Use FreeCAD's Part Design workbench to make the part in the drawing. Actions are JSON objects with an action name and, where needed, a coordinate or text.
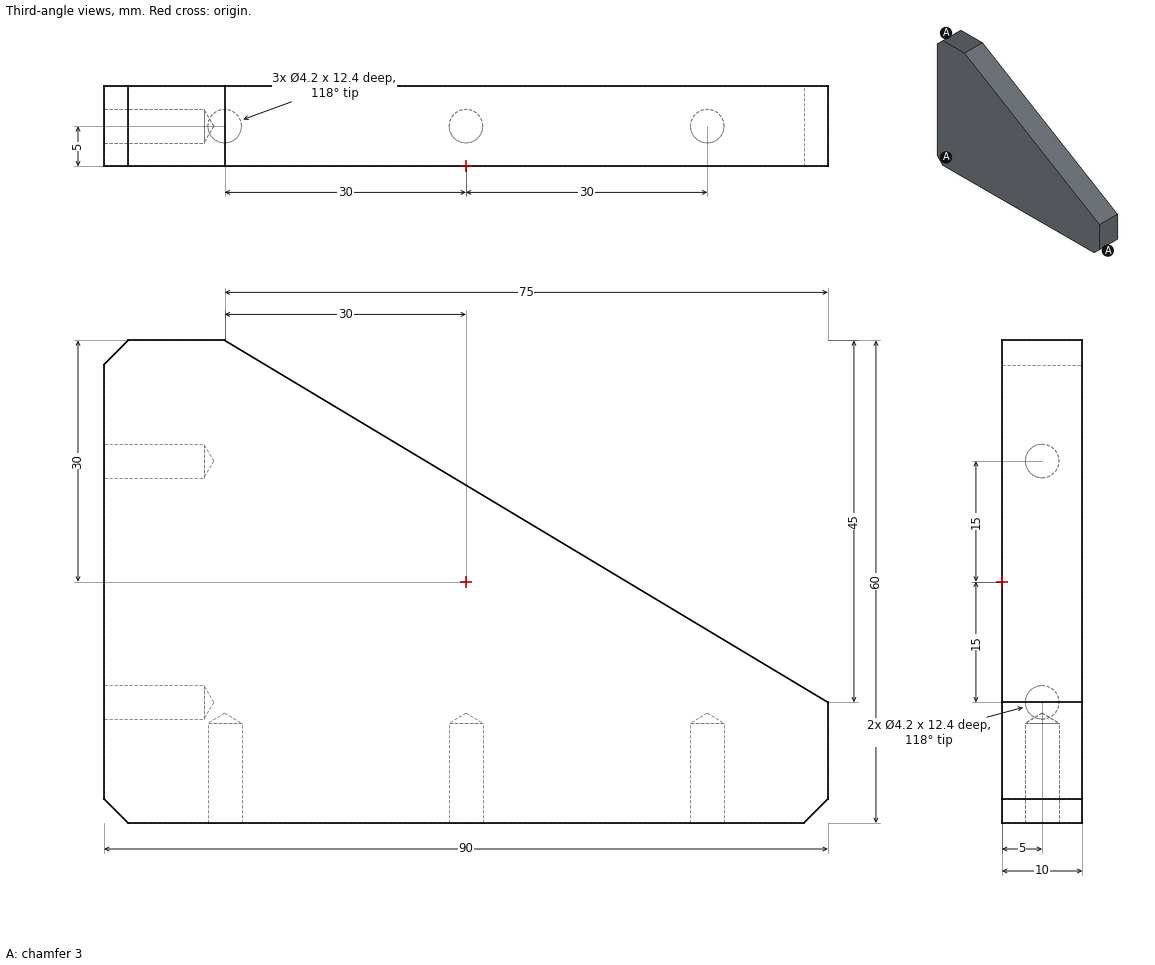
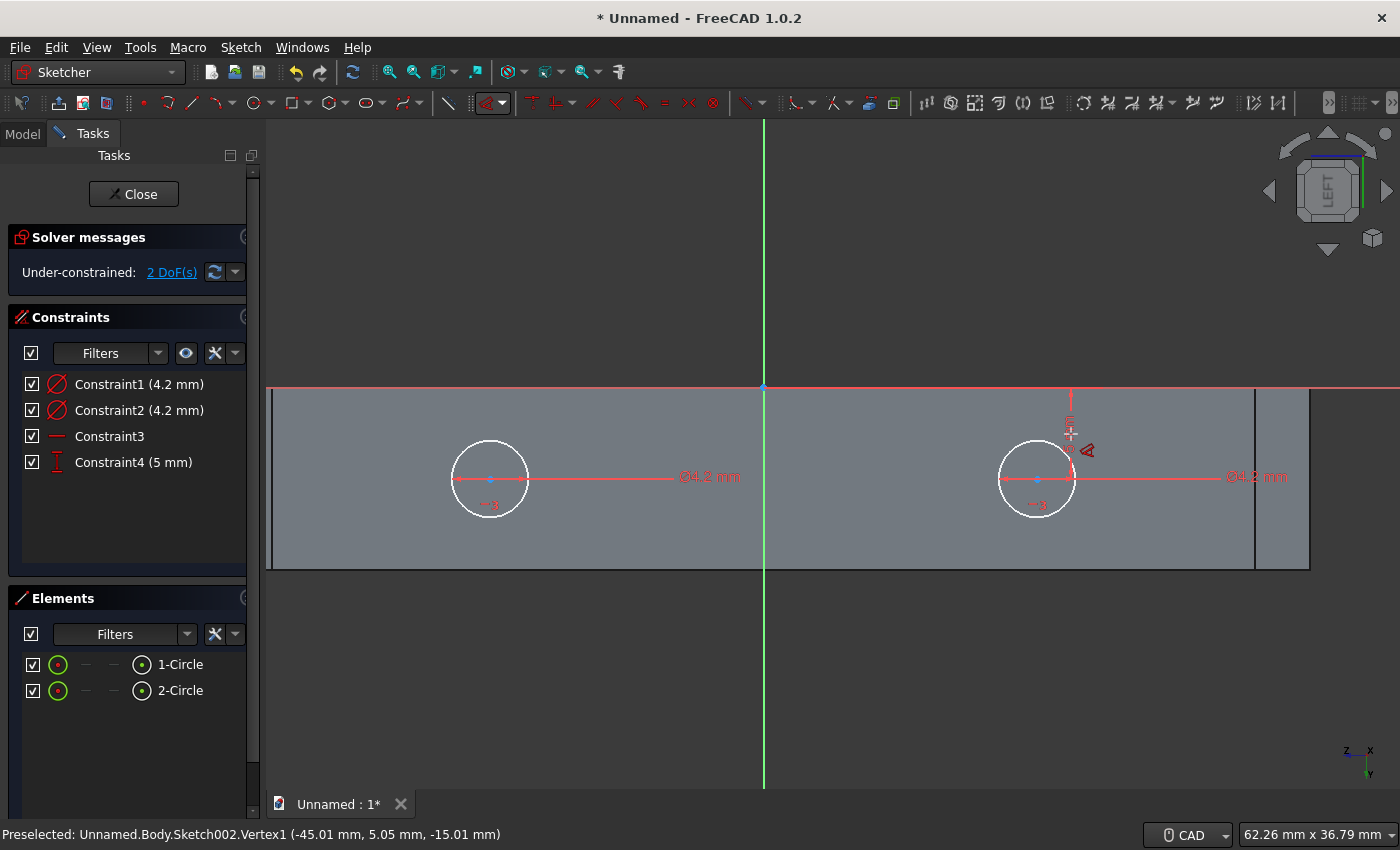
{"action": "left_click", "coordinate": [1037, 479]}
{"action": "left_click", "coordinate": [900, 354]}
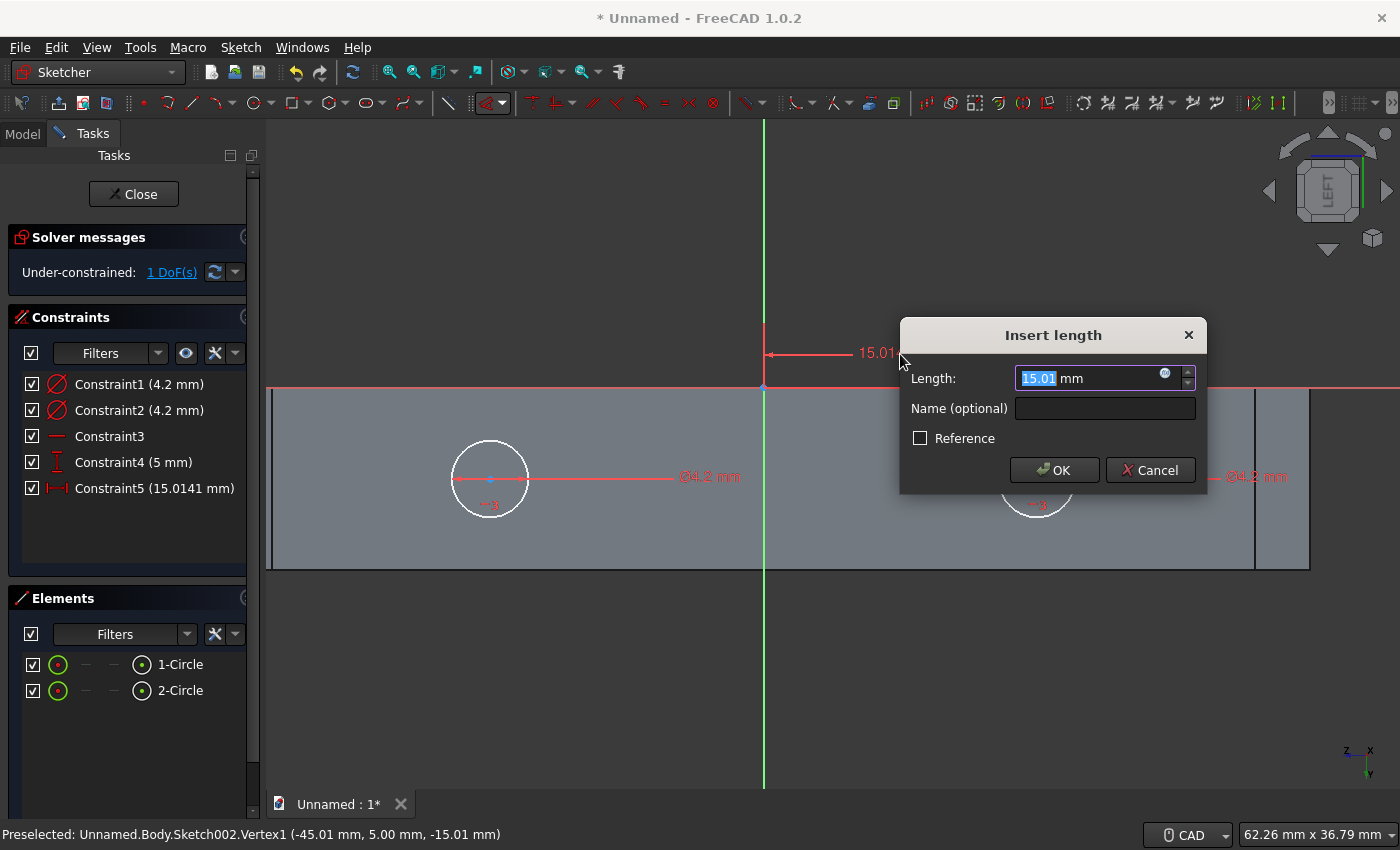
{"action": "type", "text": "15"}
{"action": "key", "text": "Return"}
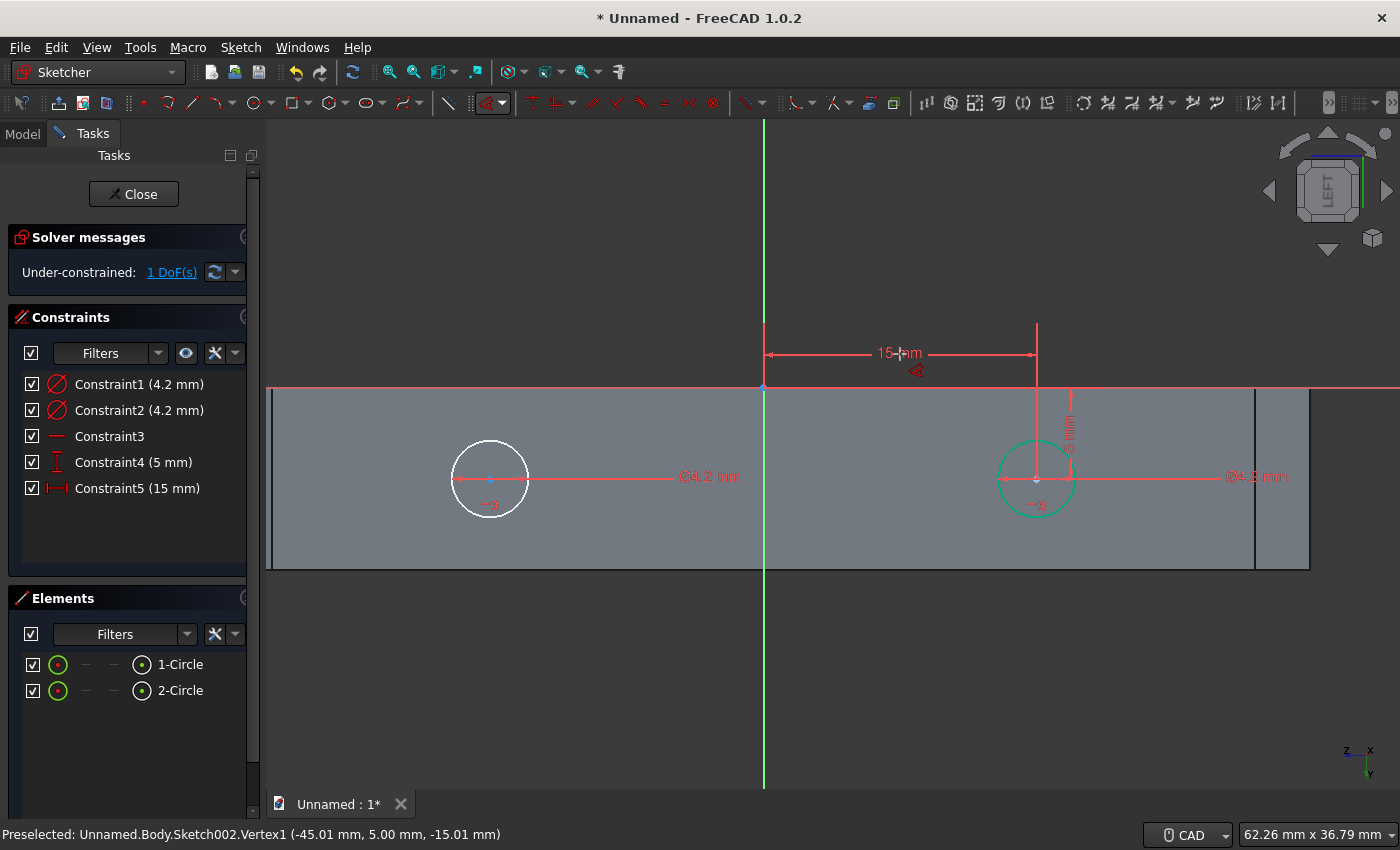
{"action": "left_click", "coordinate": [490, 479]}
{"action": "left_click", "coordinate": [627, 354]}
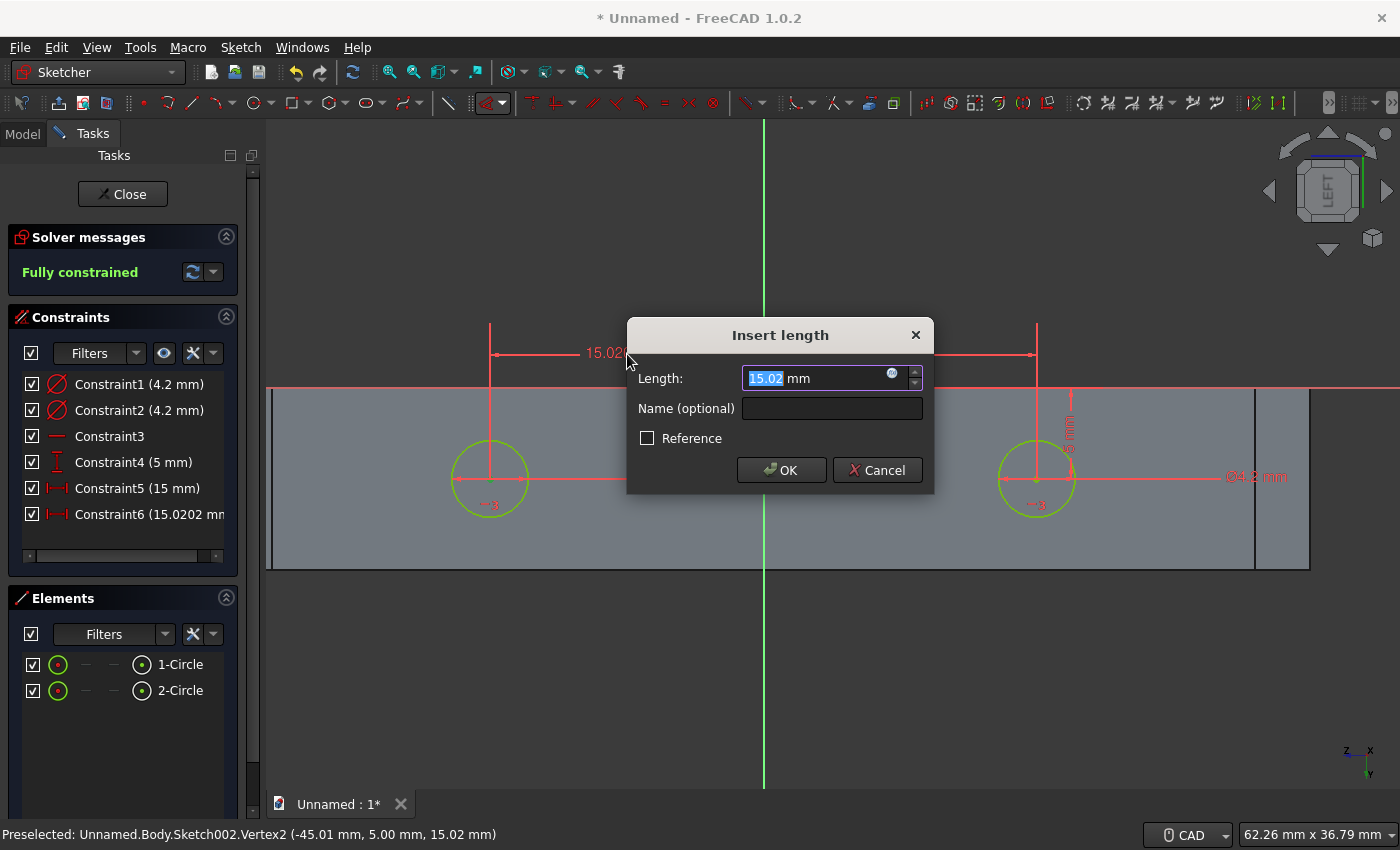
{"action": "type", "text": "15"}
{"action": "key", "text": "Return"}
{"action": "key", "text": "Escape"}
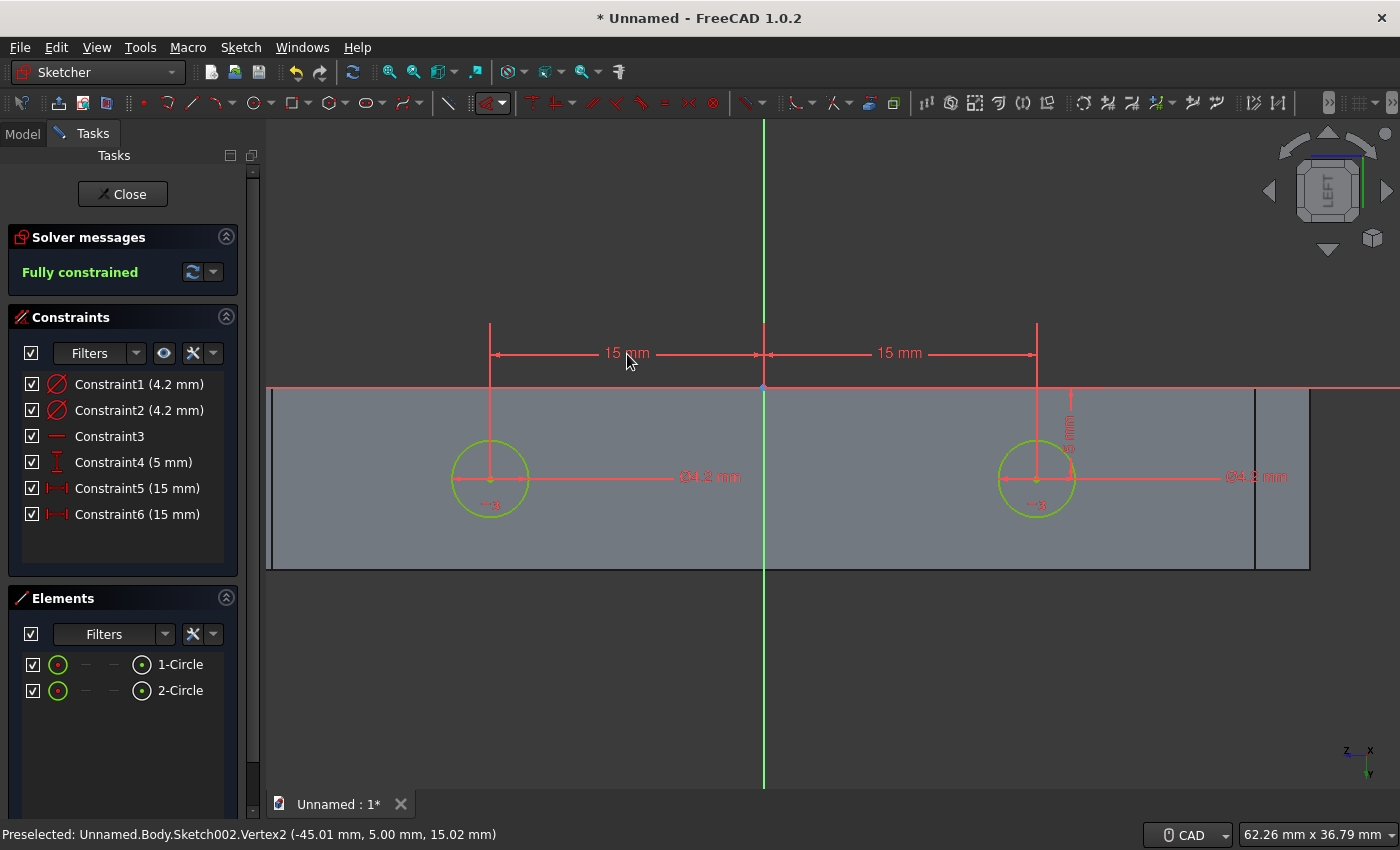
{"action": "left_click", "coordinate": [123, 194]}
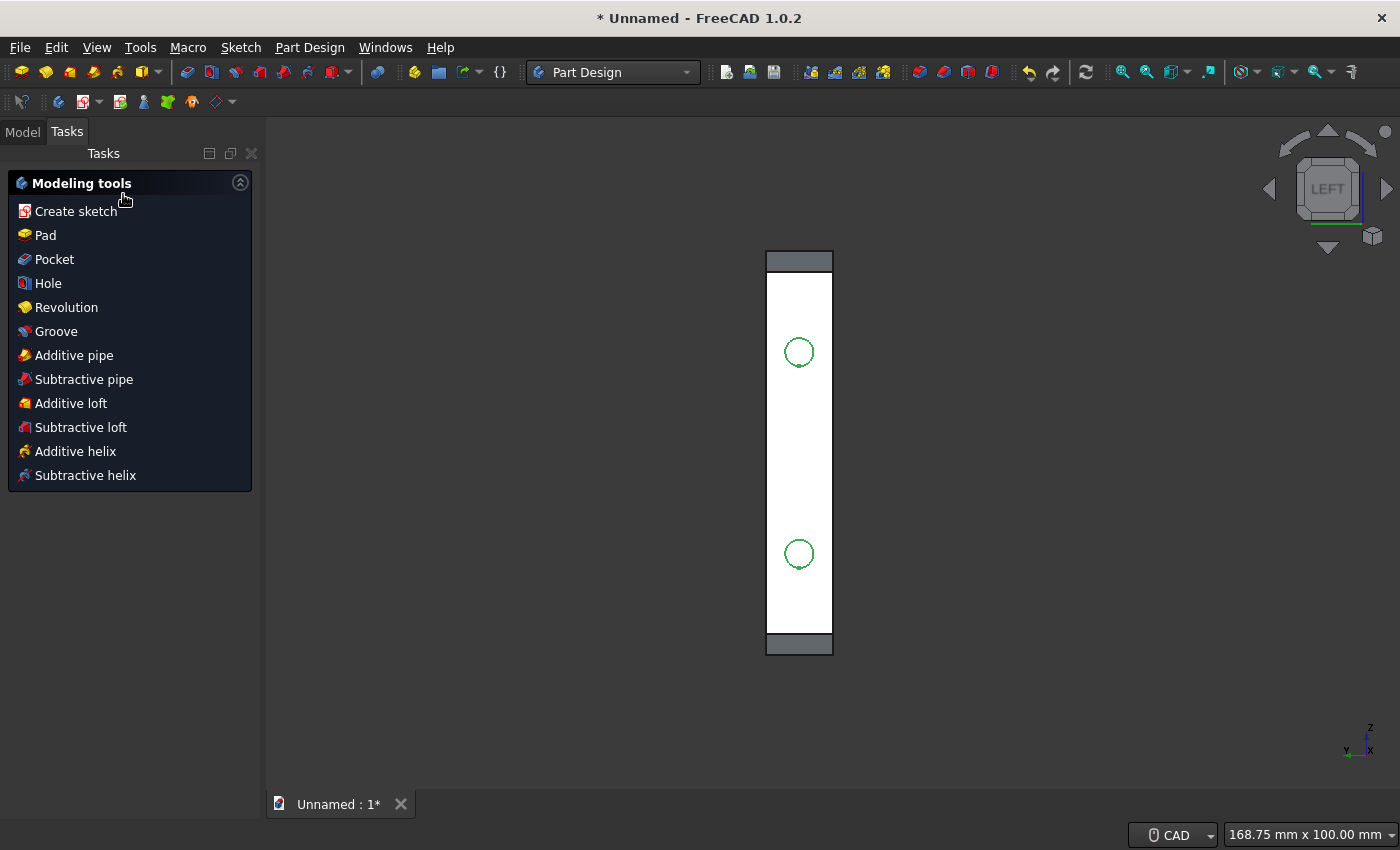
{"action": "left_click", "coordinate": [212, 72]}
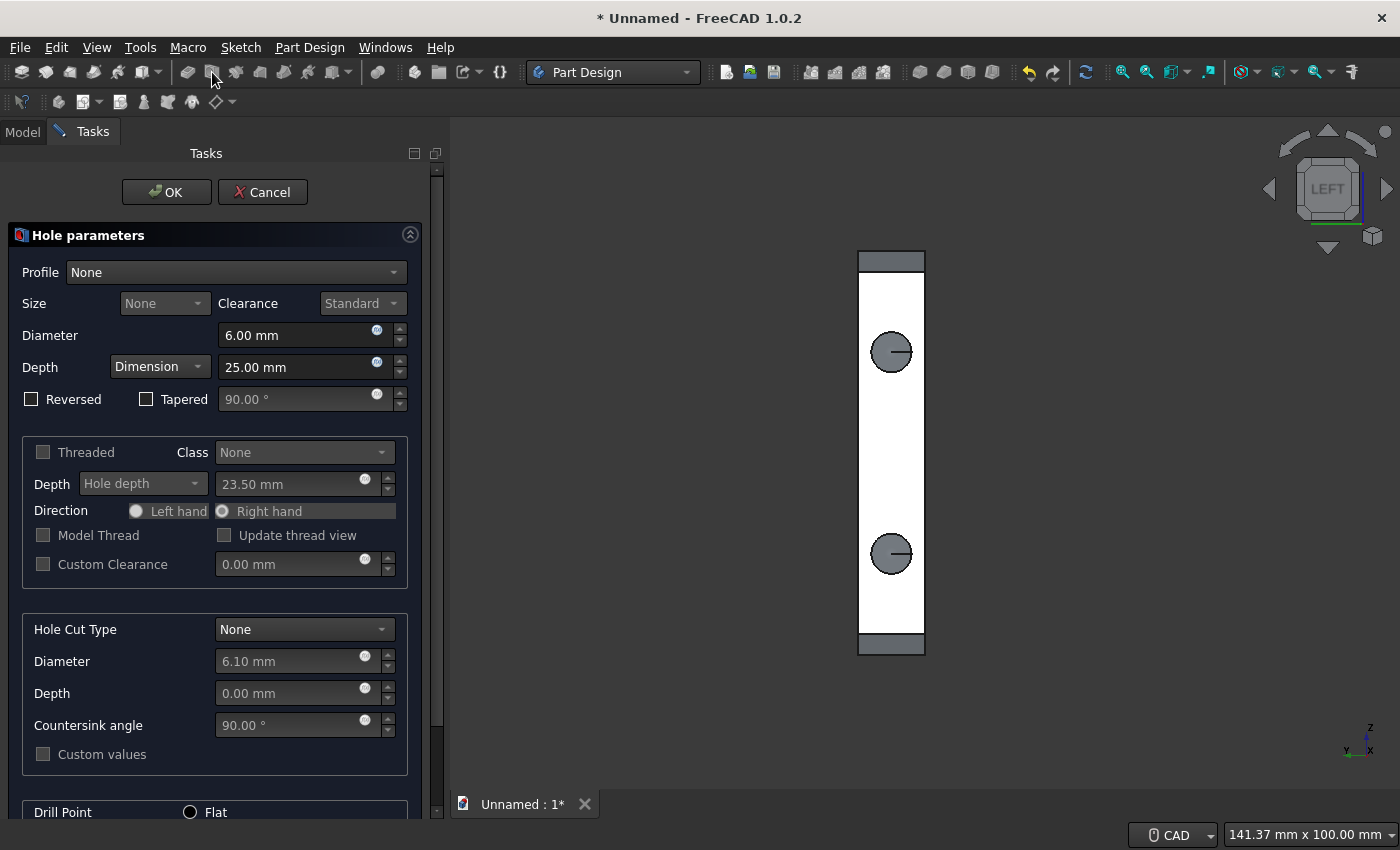
{"action": "triple_click", "coordinate": [305, 335]}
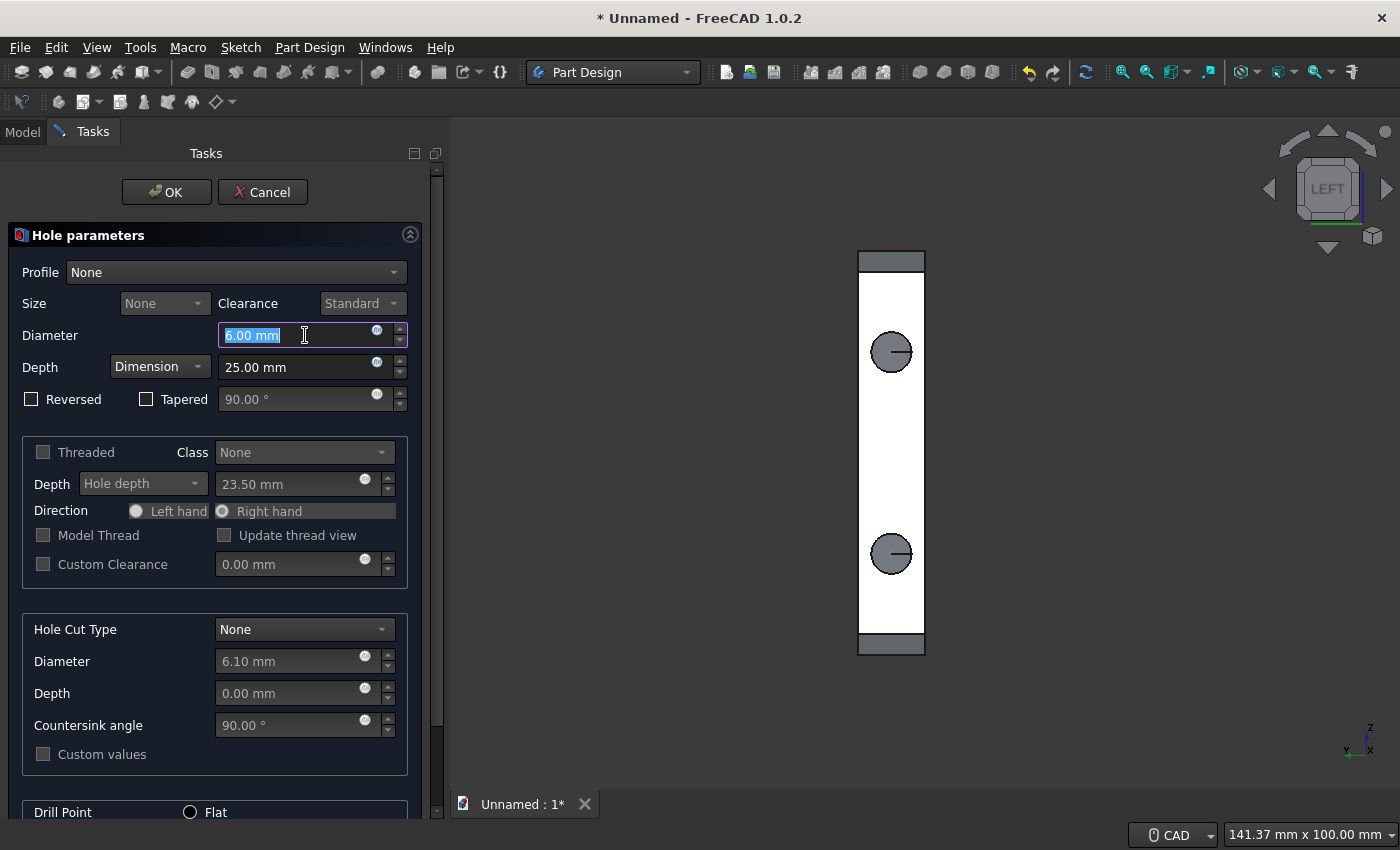
{"action": "type", "text": "4.2"}
{"action": "key", "text": "Tab"}